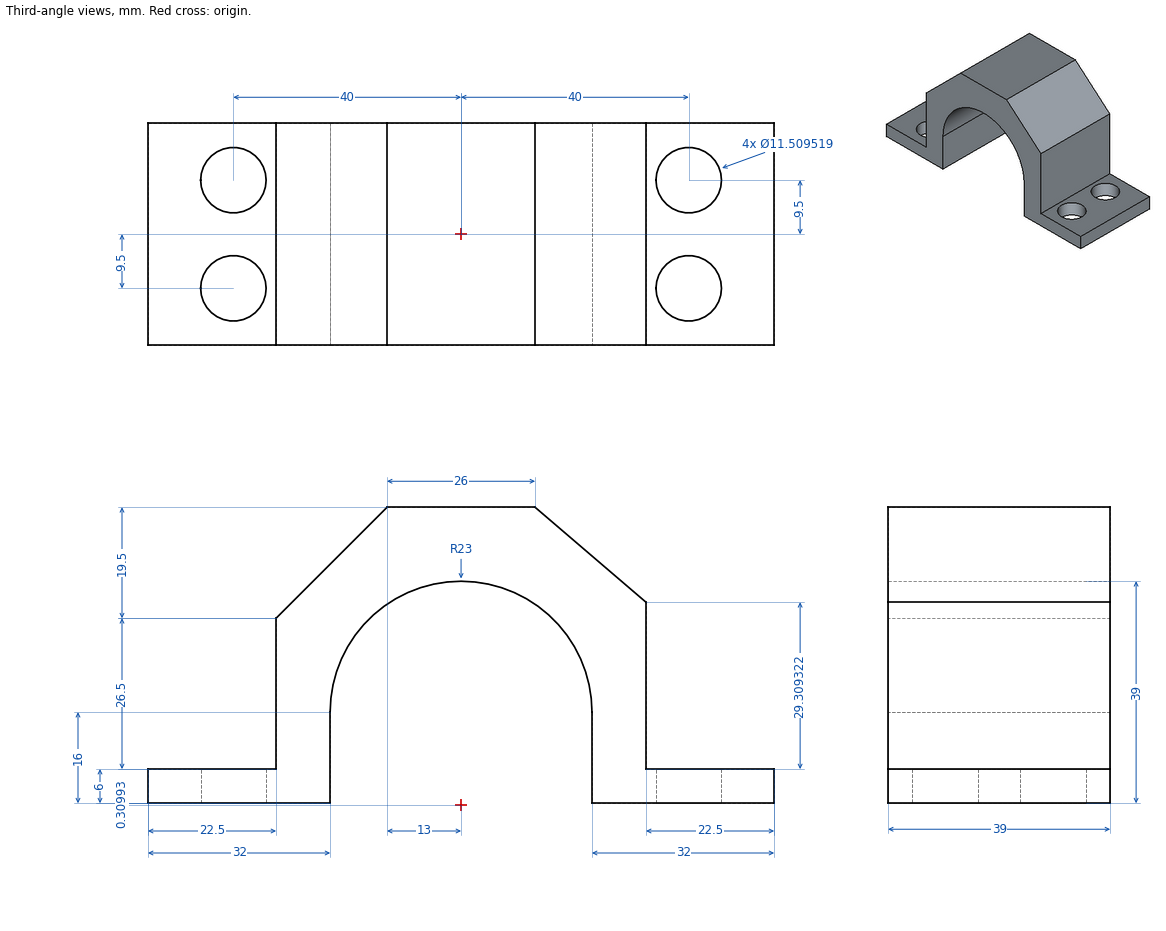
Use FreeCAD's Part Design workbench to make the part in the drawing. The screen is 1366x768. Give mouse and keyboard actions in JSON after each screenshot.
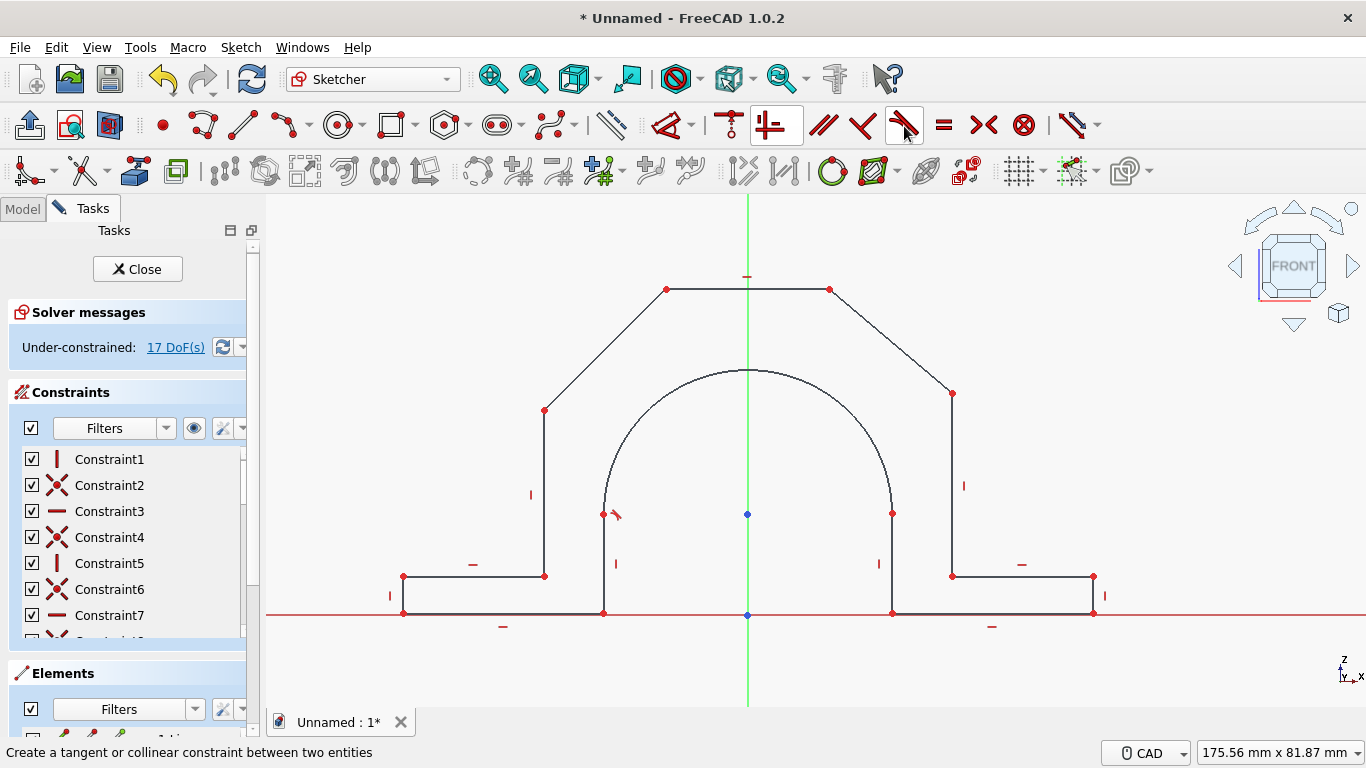
{"action": "left_click", "coordinate": [892, 584]}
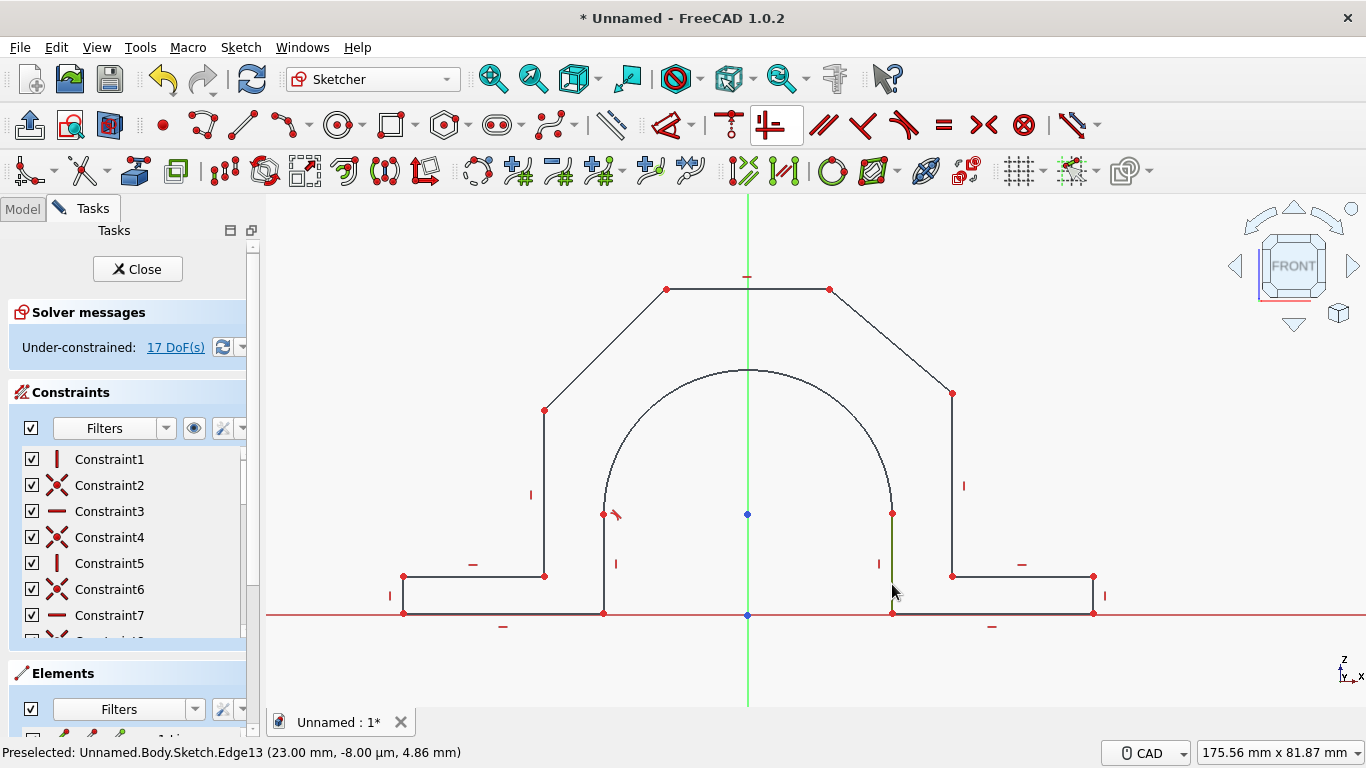
{"action": "left_click", "coordinate": [833, 398]}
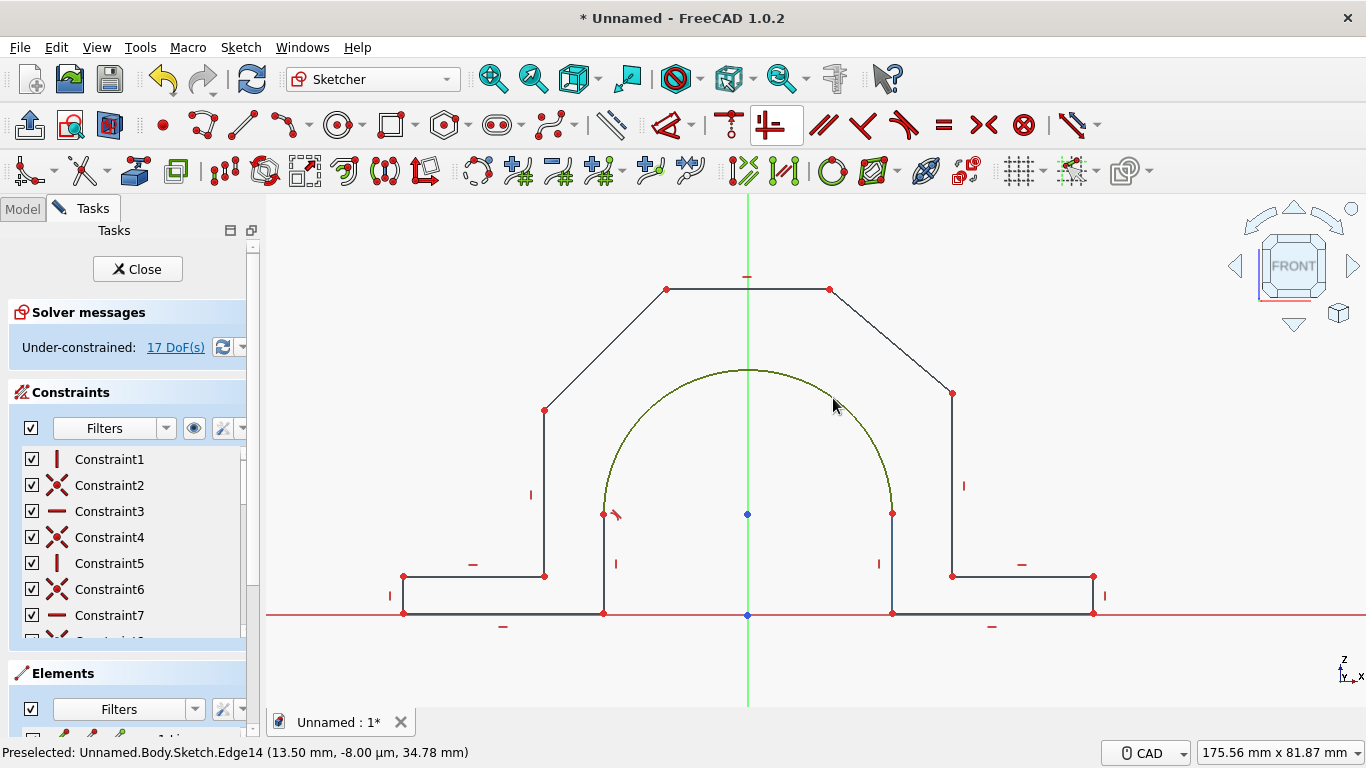
{"action": "key", "text": "t"}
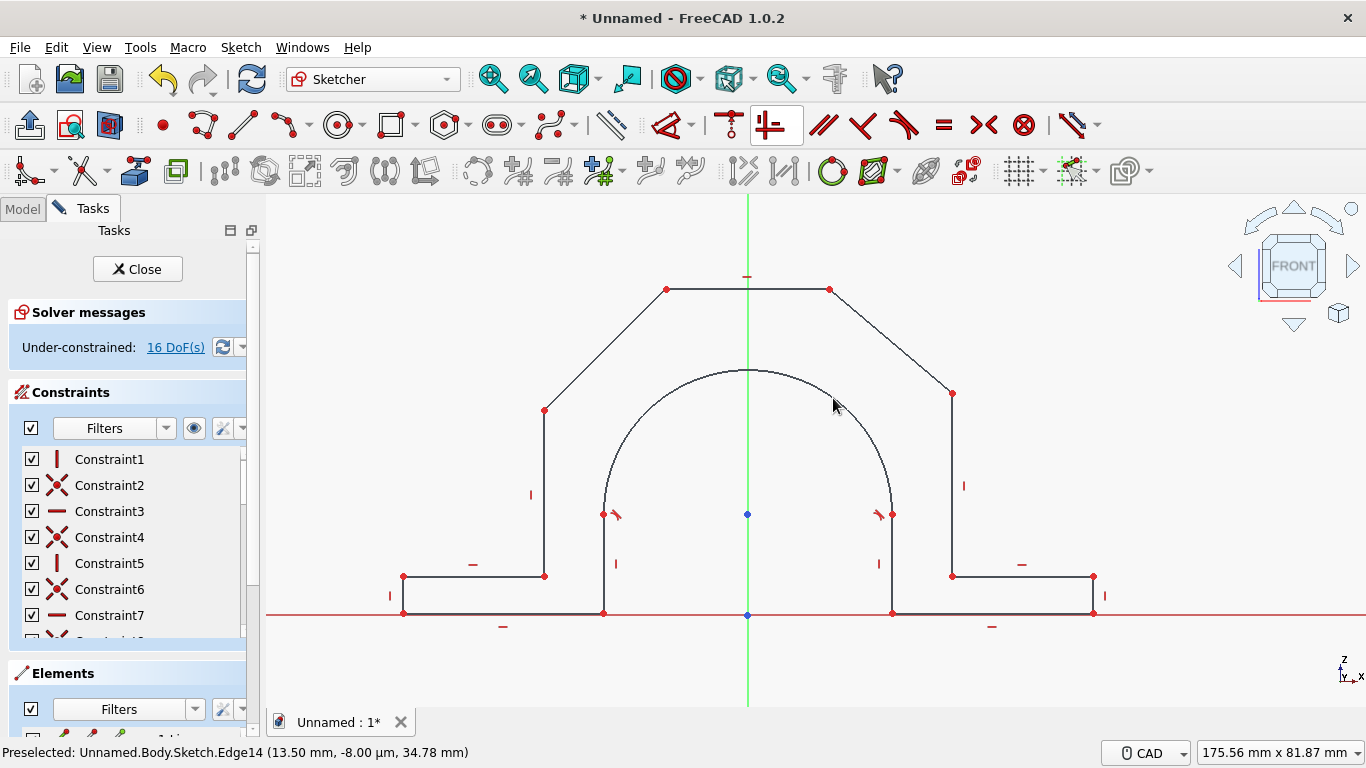
{"action": "left_click", "coordinate": [748, 514]}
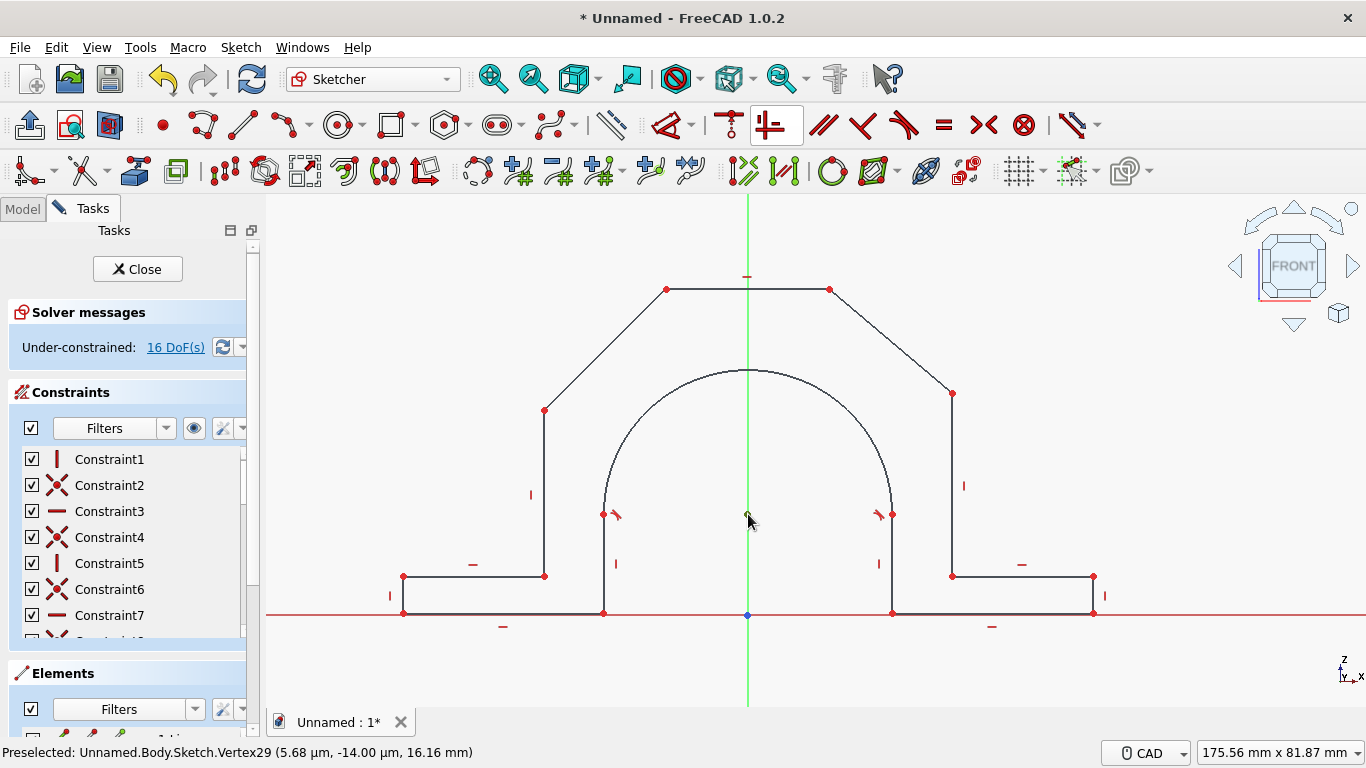
{"action": "left_click", "coordinate": [748, 646]}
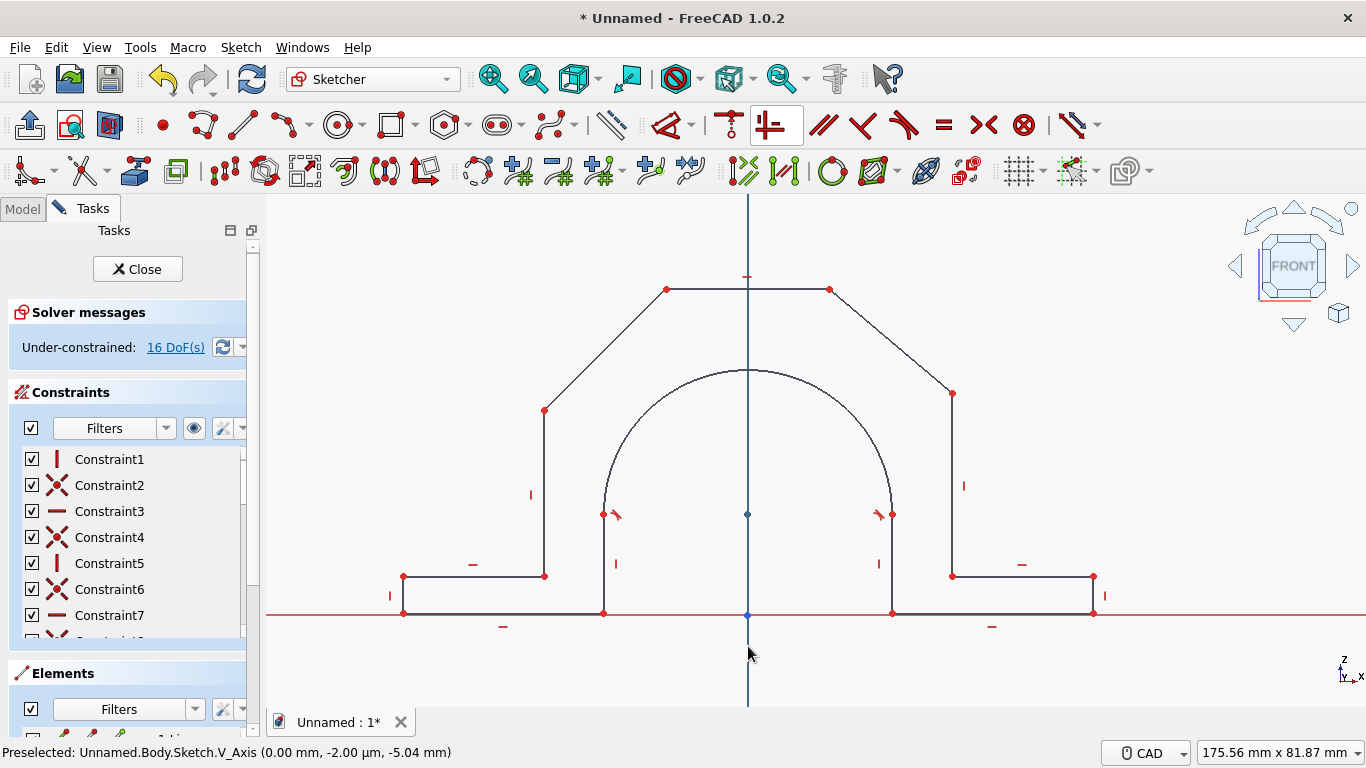
{"action": "key", "text": "c"}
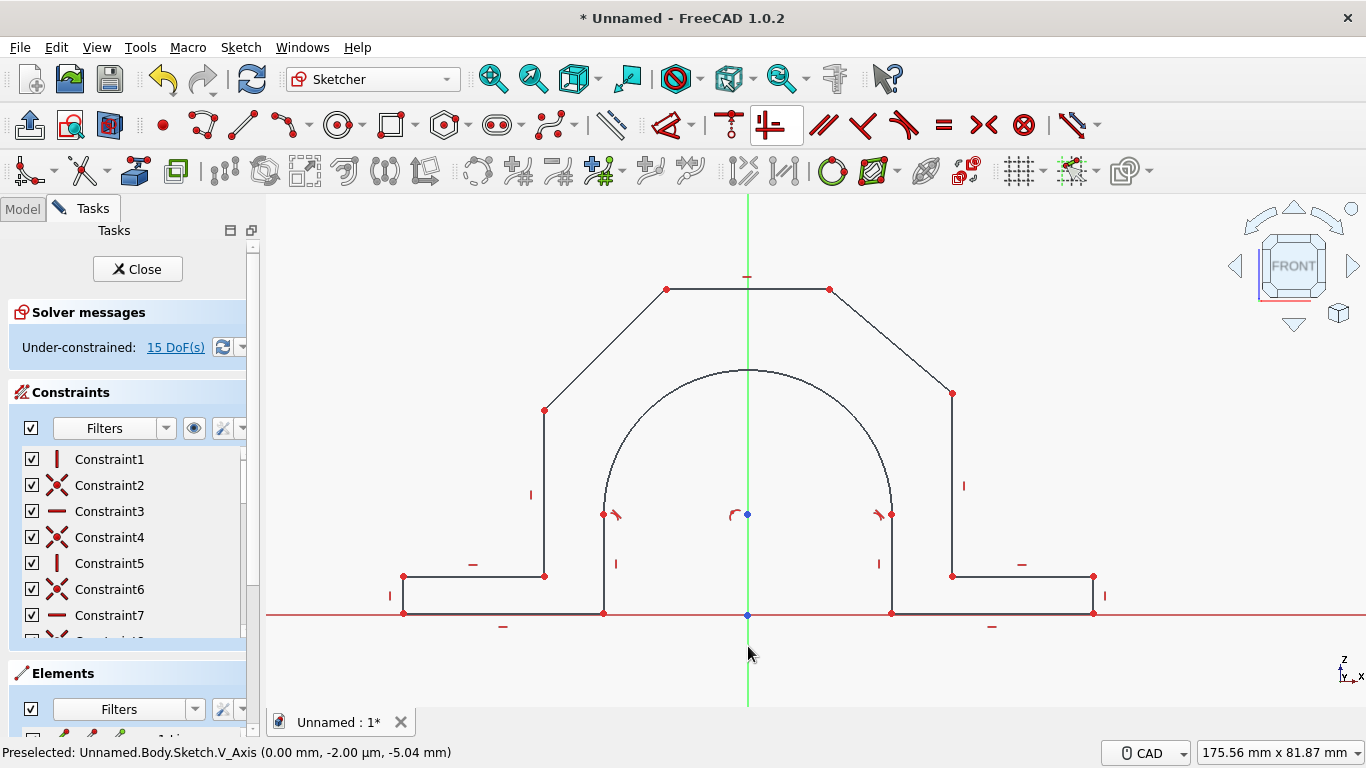
{"action": "key", "text": "d"}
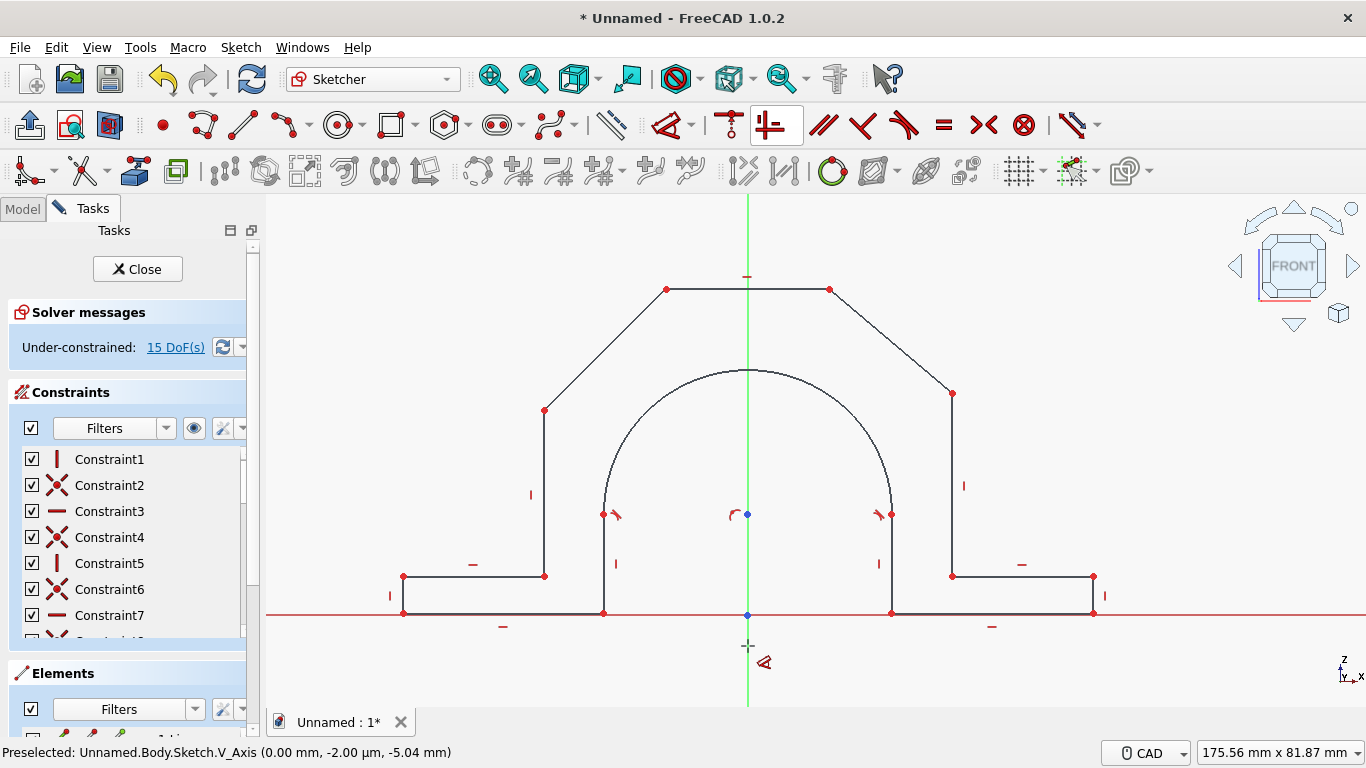
{"action": "left_click", "coordinate": [833, 398]}
{"action": "left_click", "coordinate": [852, 372]}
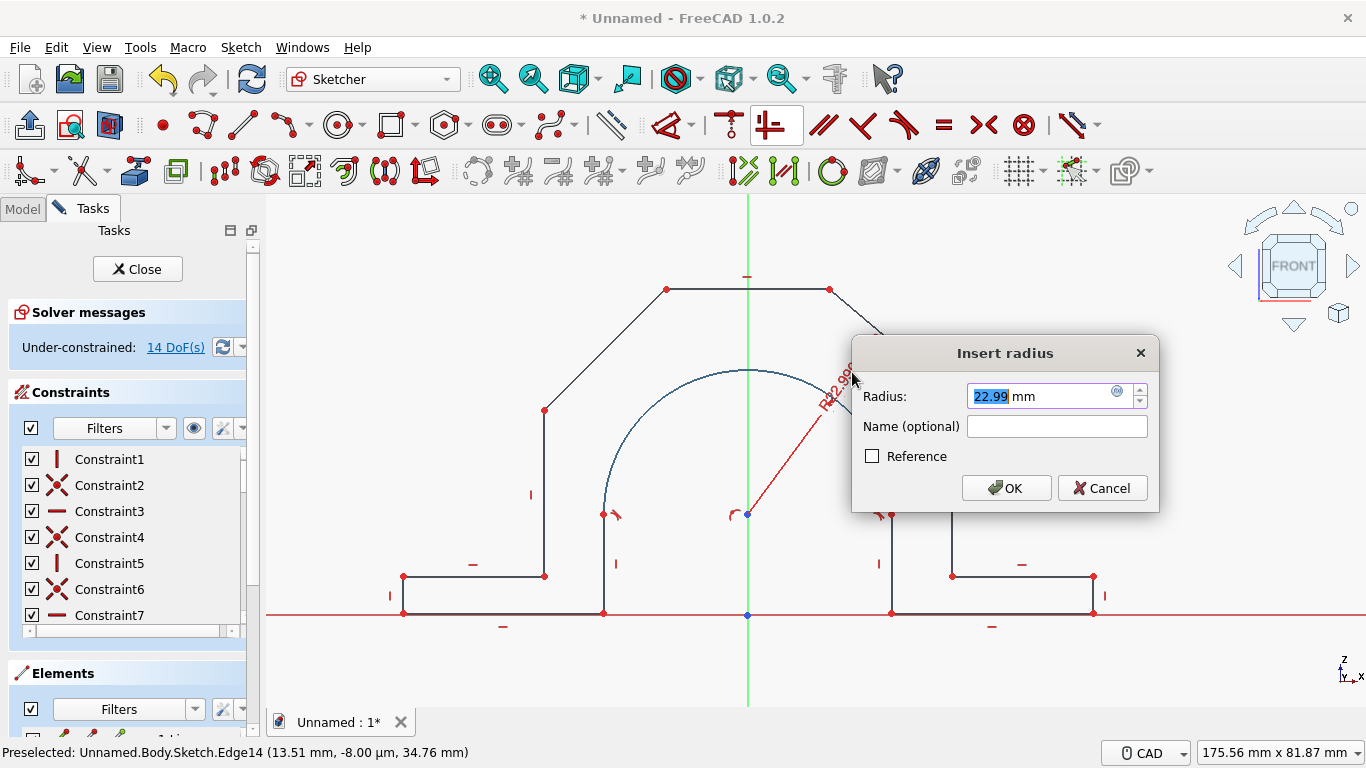
{"action": "type", "text": "23"}
{"action": "key", "text": "Return"}